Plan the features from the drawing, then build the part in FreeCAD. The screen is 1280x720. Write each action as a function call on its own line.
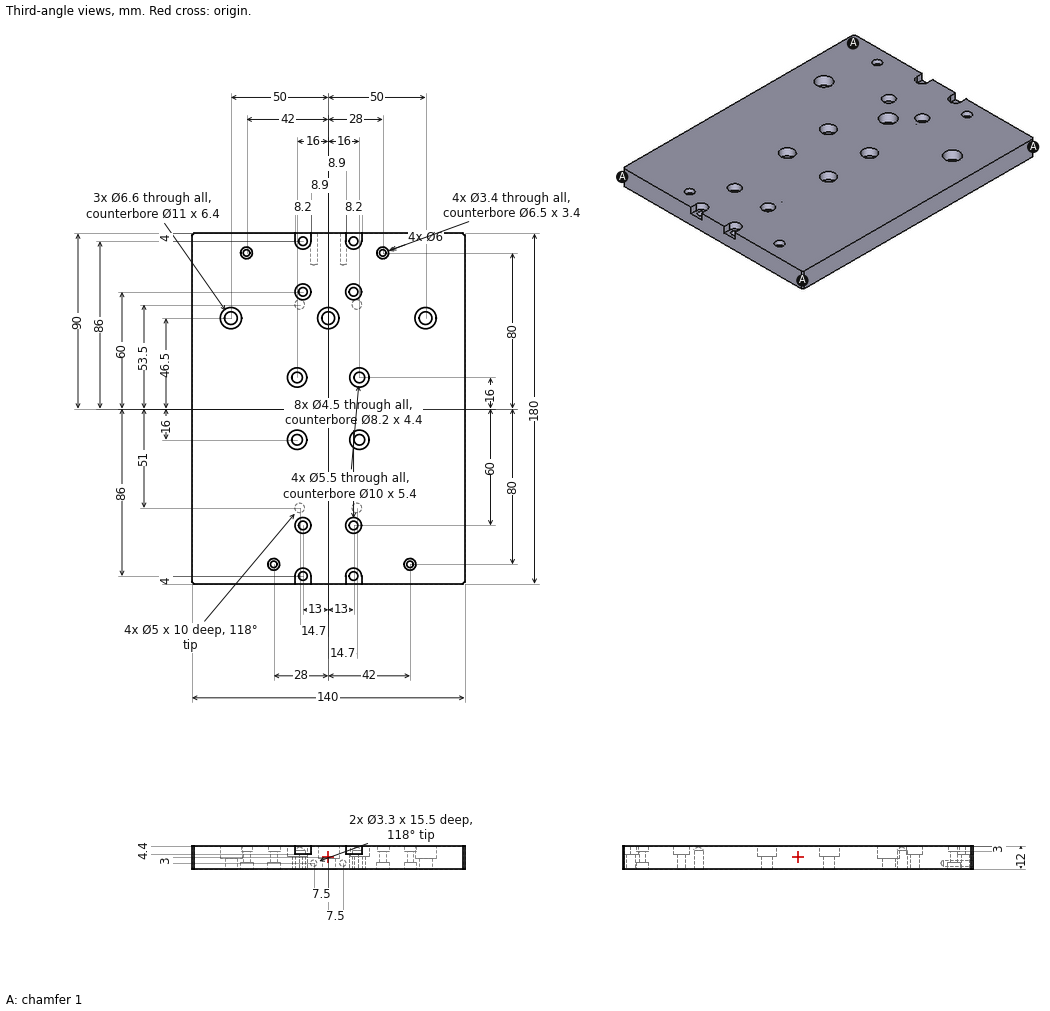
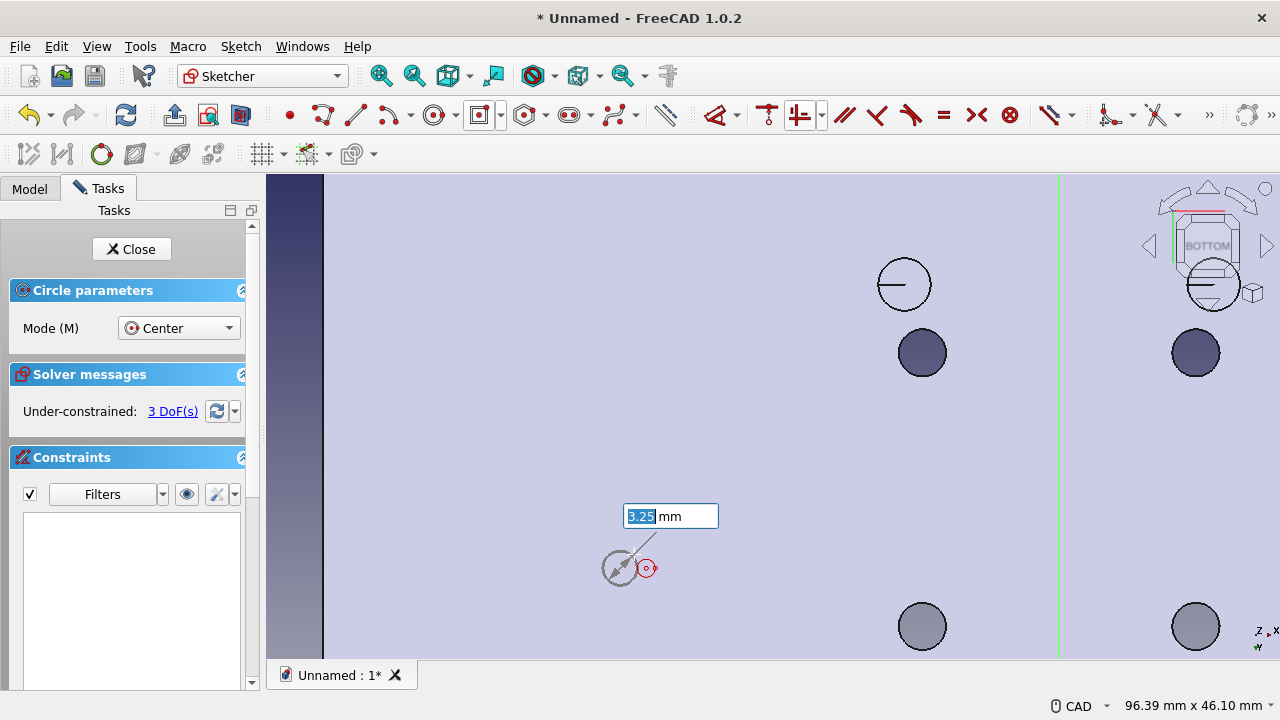
click(630, 551)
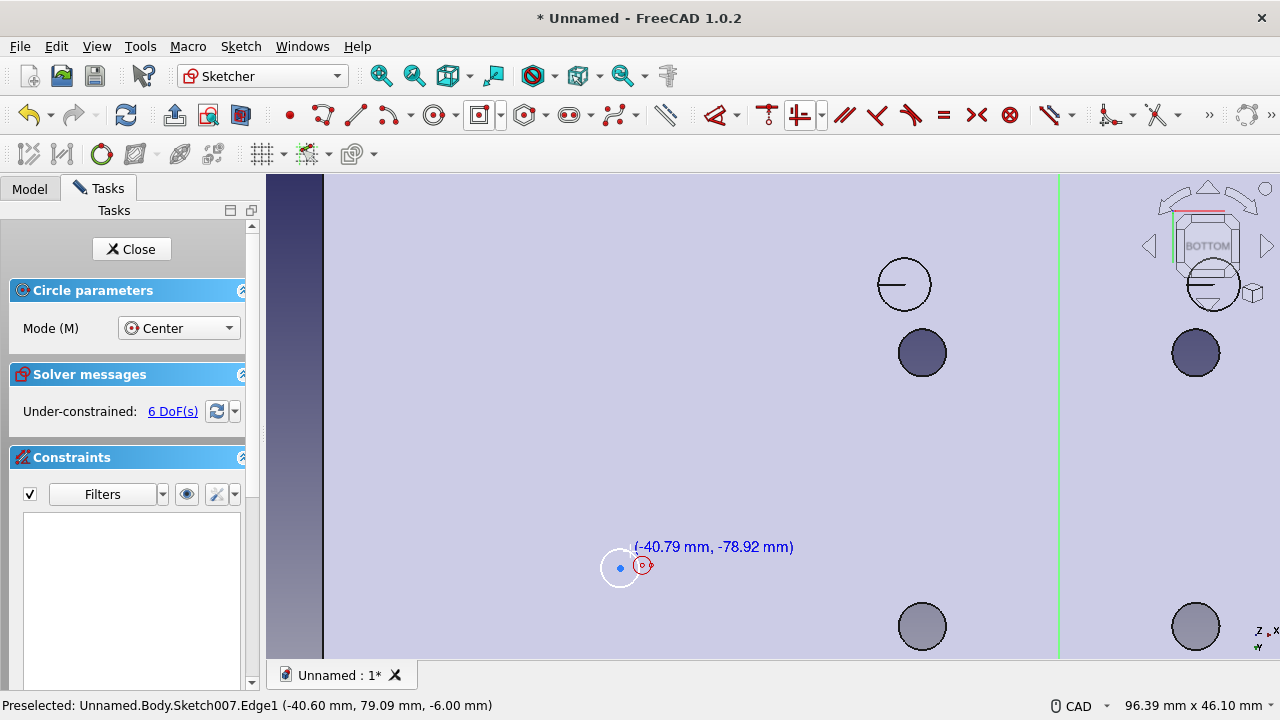
scroll(634, 554, down, 9)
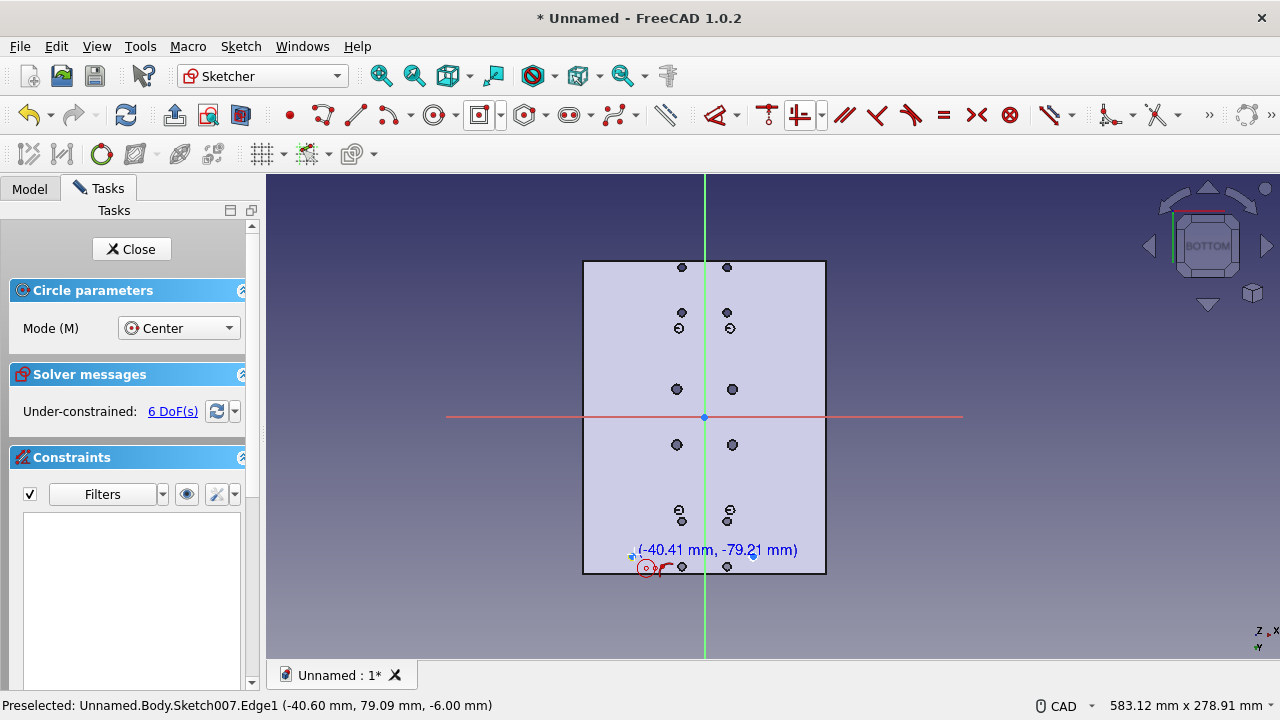
scroll(656, 278, up, 11)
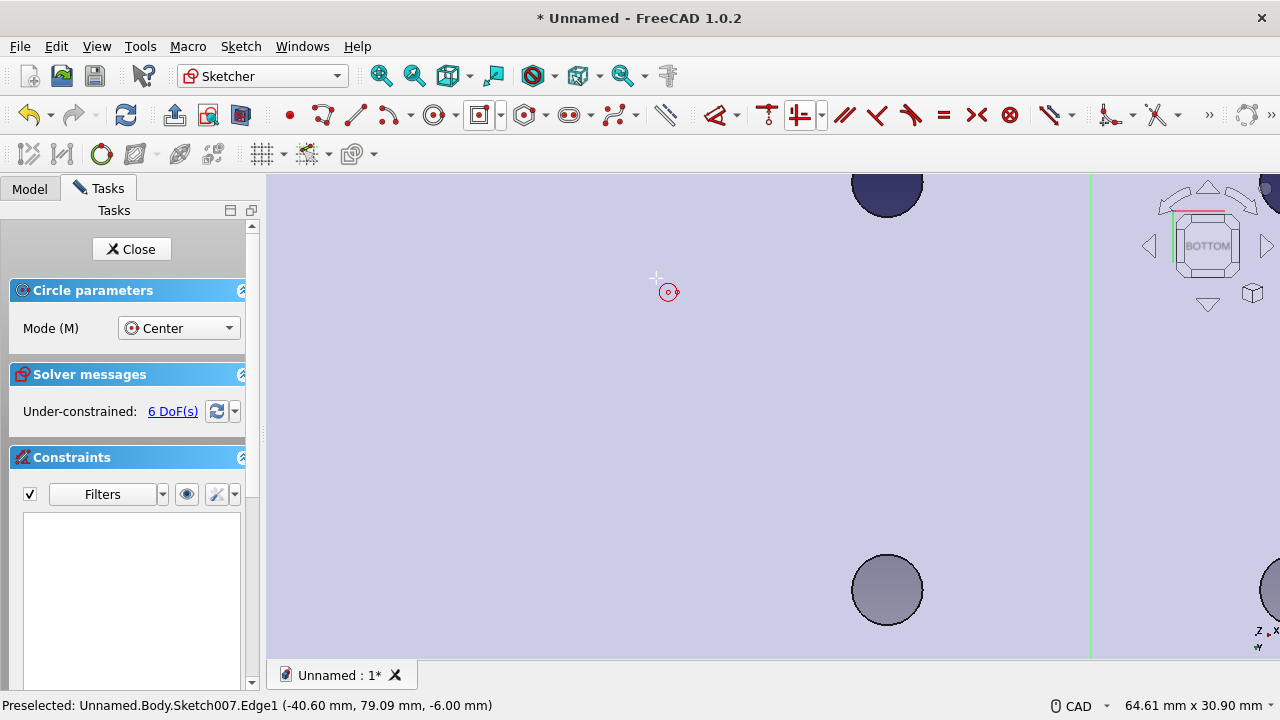
scroll(656, 278, down, 11)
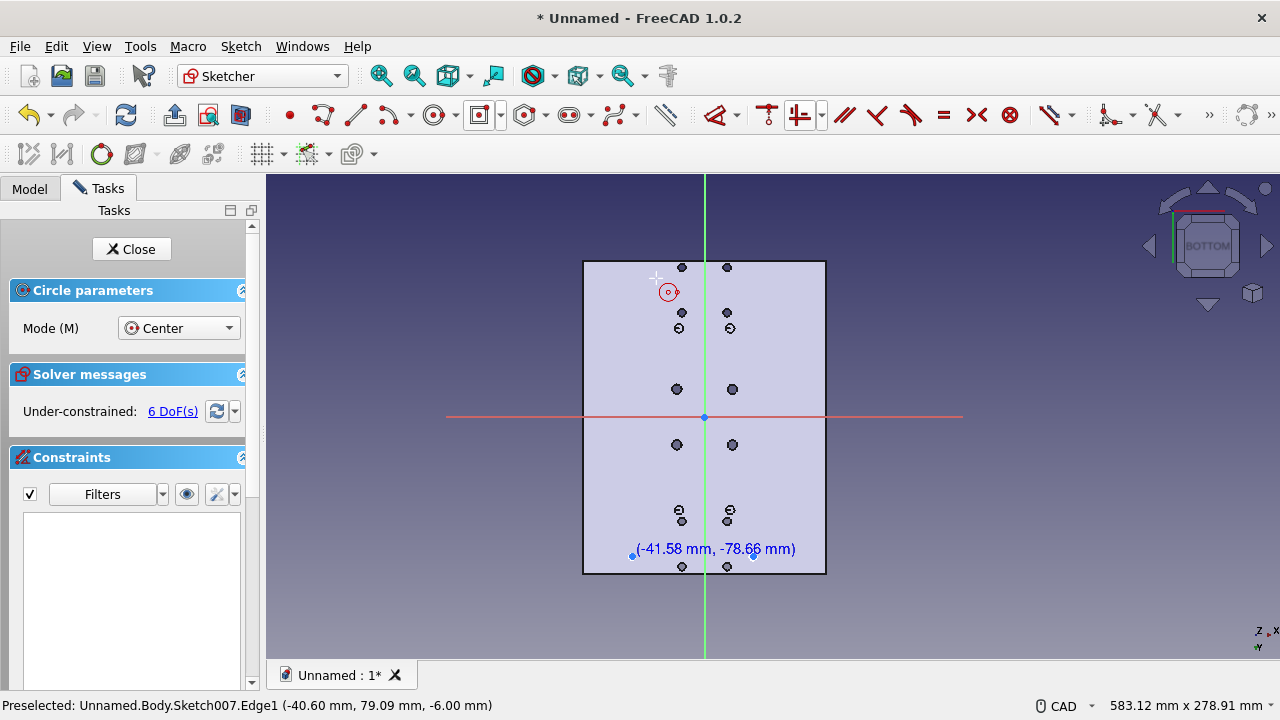
click(656, 278)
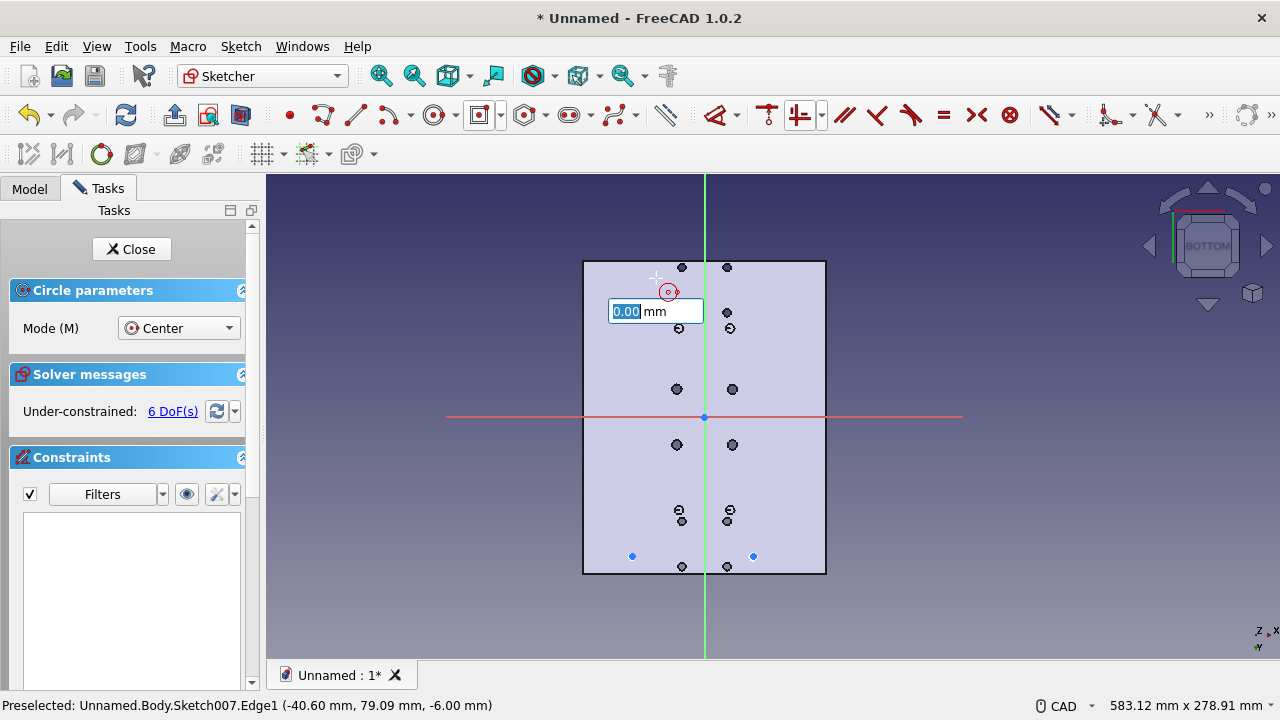
scroll(658, 276, up, 9)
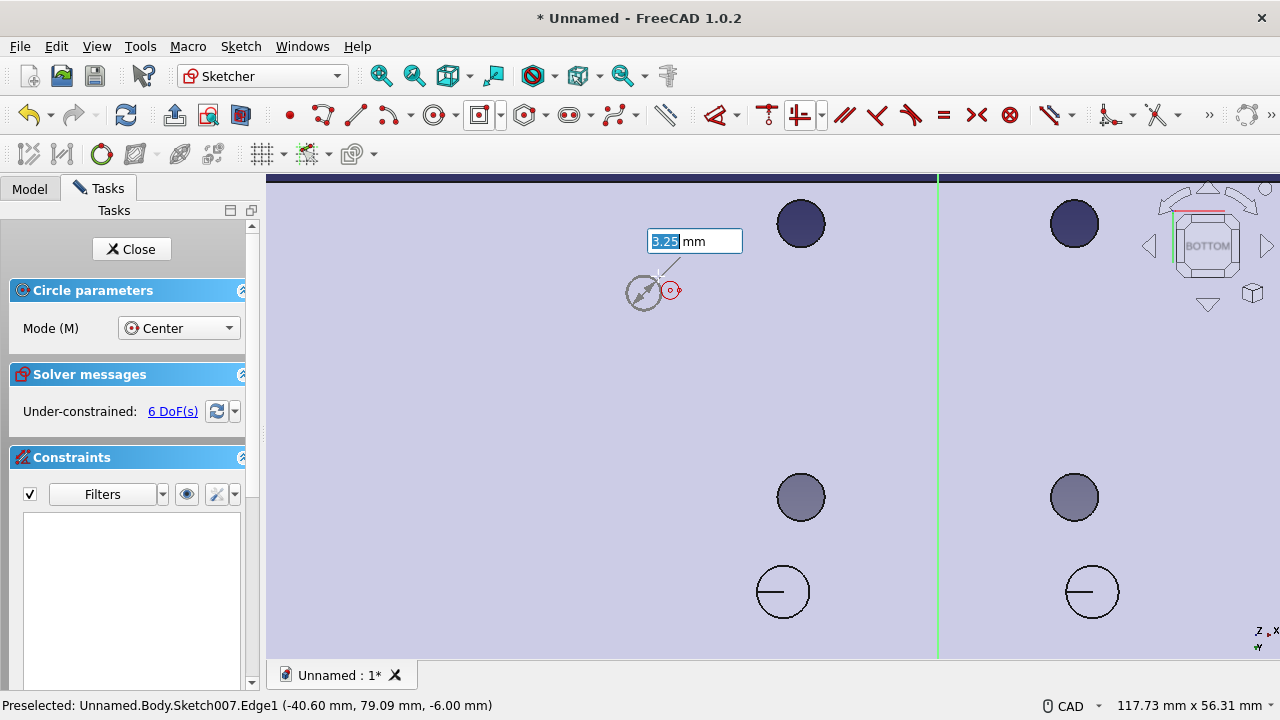
click(656, 274)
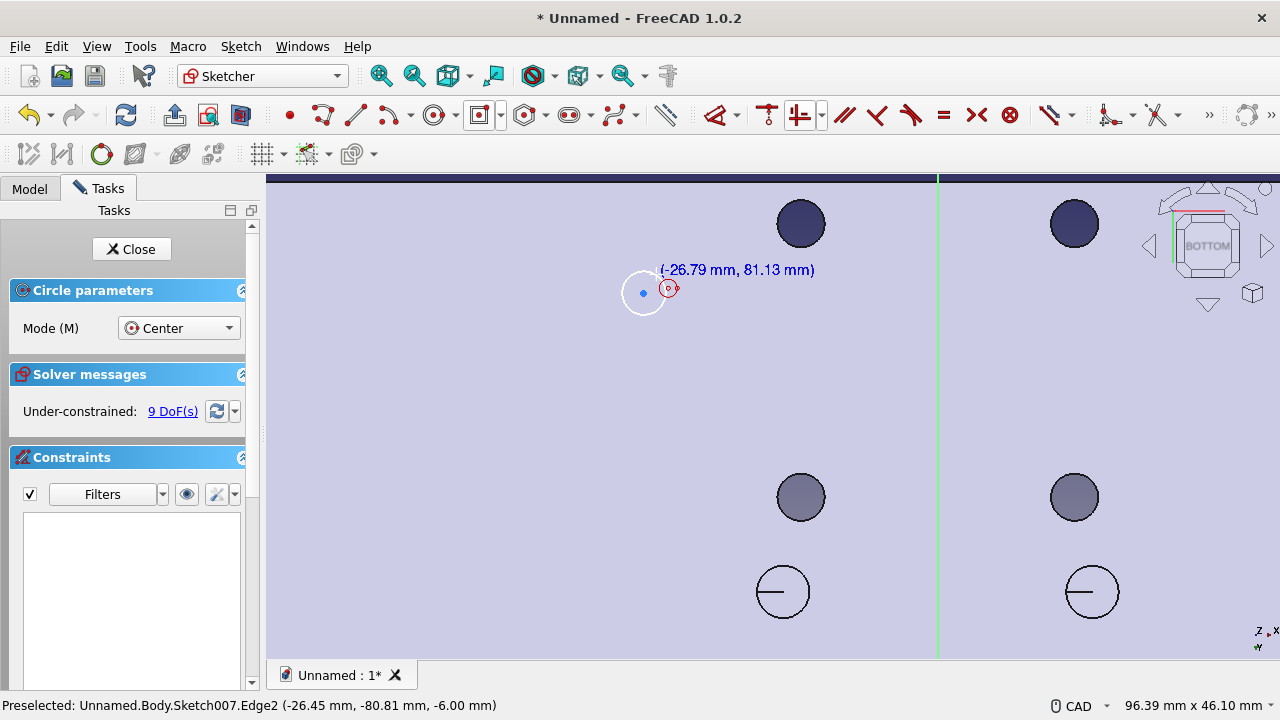
scroll(658, 276, down, 9)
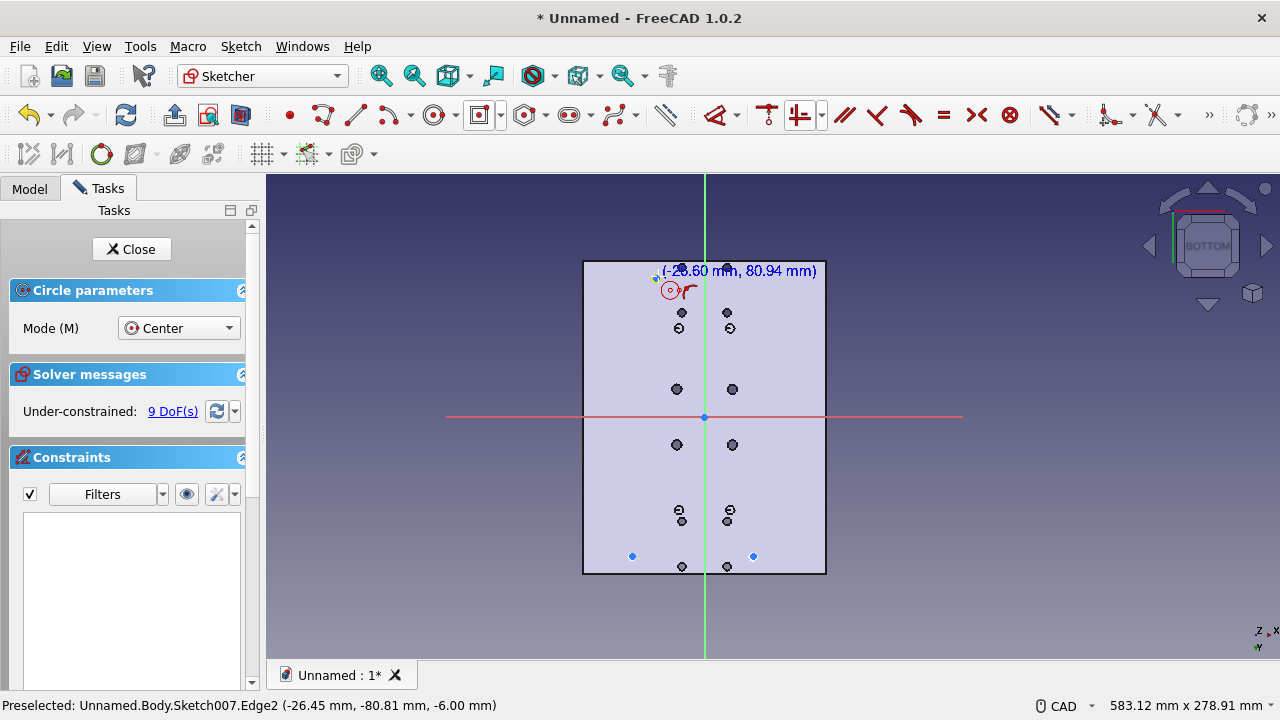
scroll(778, 278, up, 11)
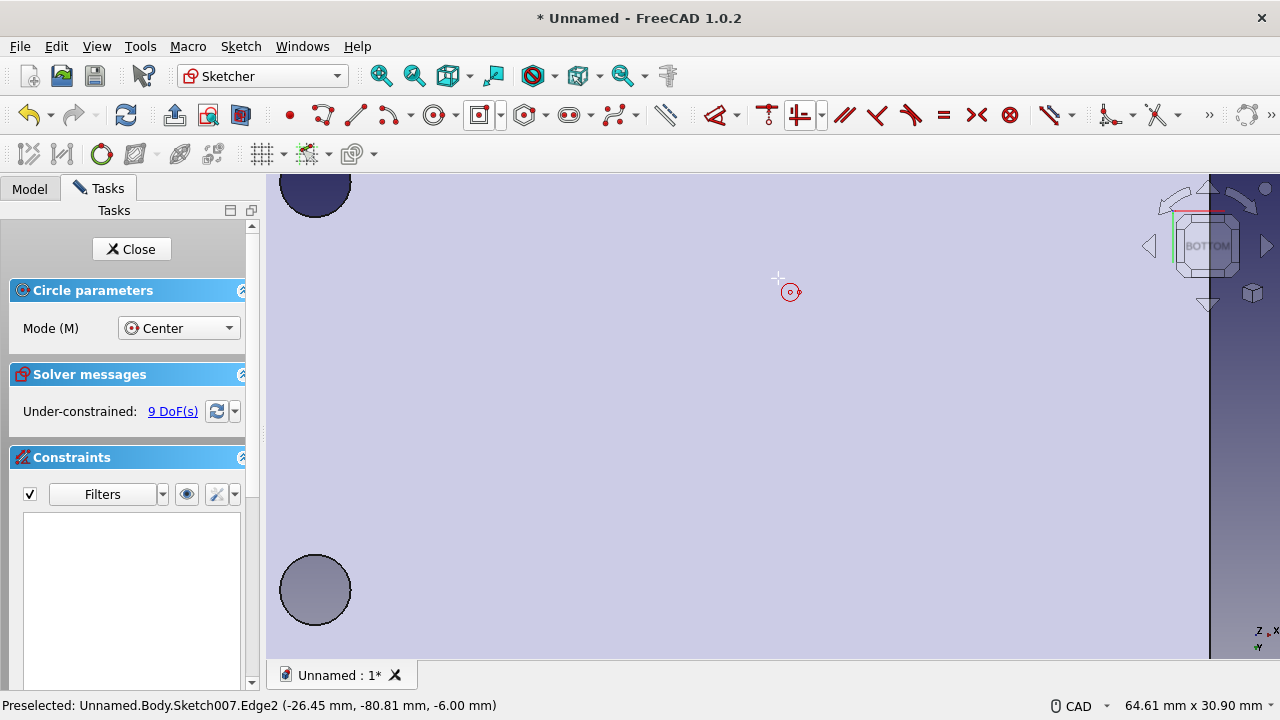
scroll(778, 278, down, 11)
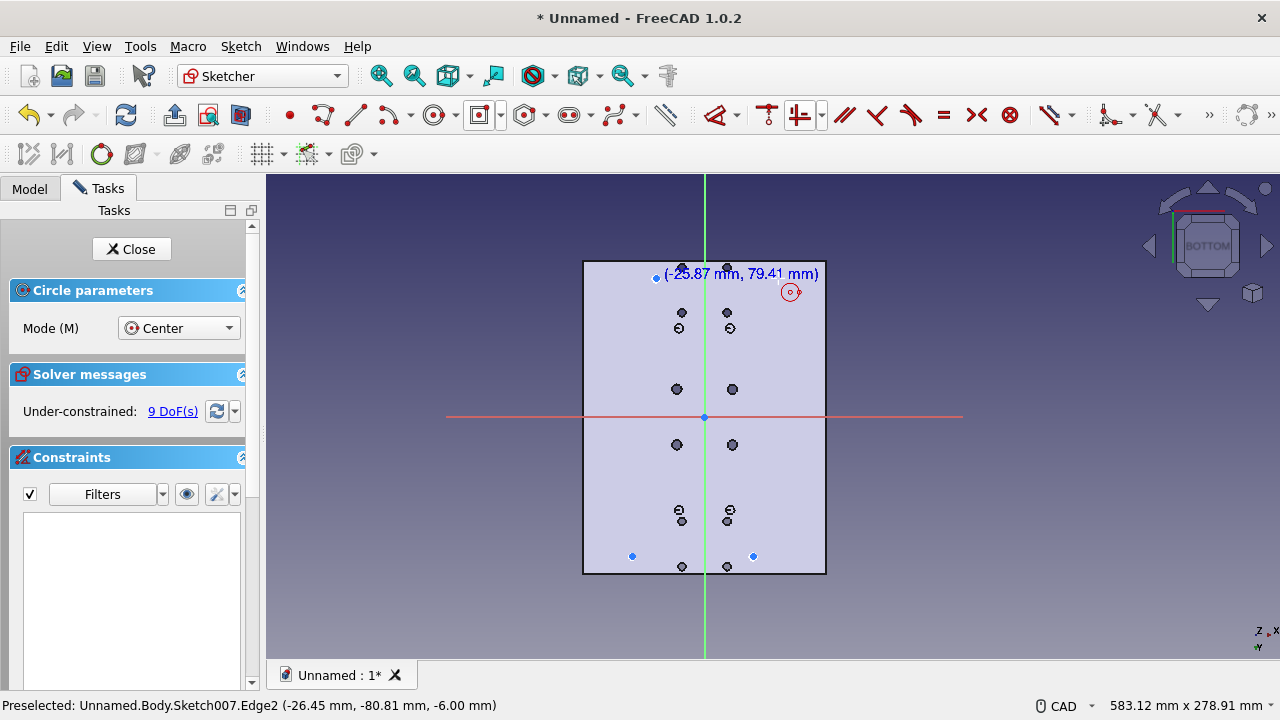
click(778, 278)